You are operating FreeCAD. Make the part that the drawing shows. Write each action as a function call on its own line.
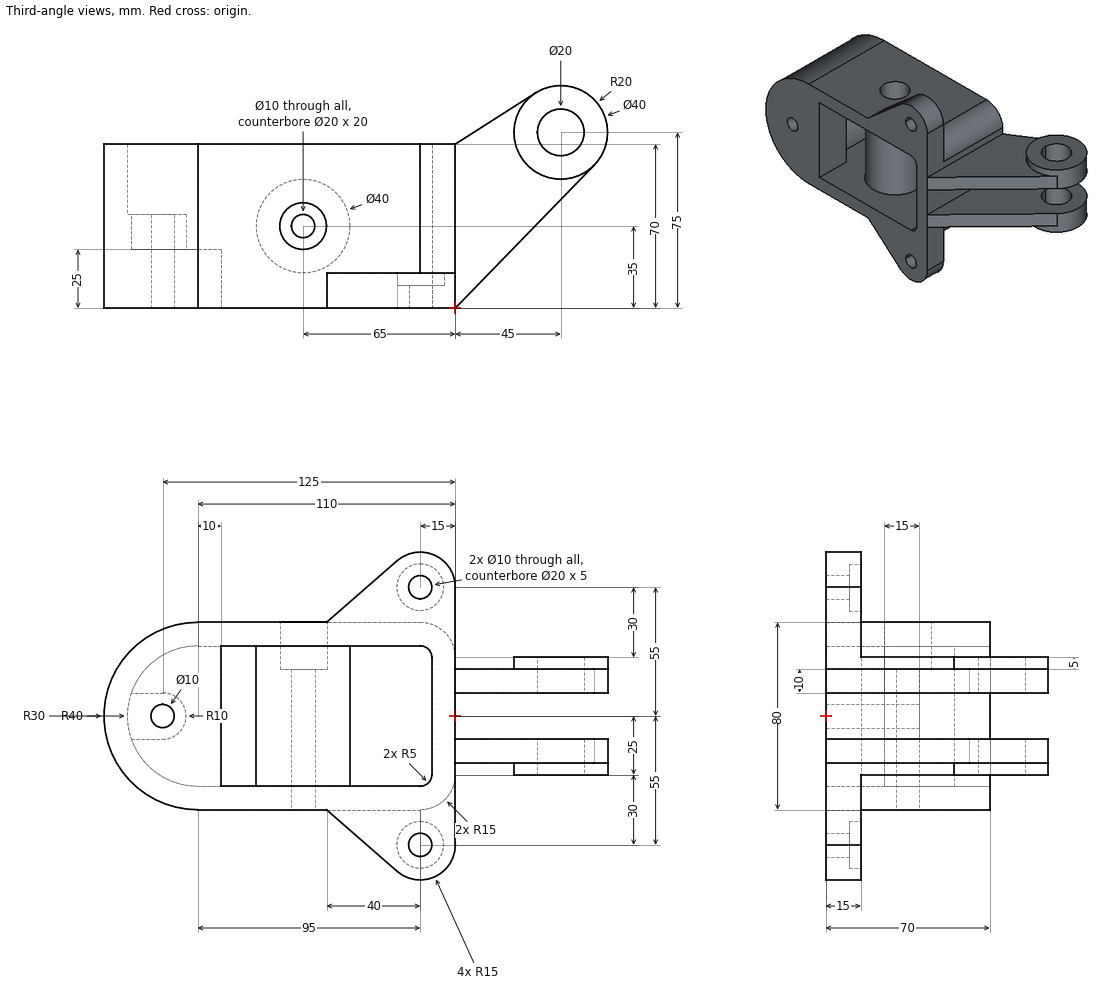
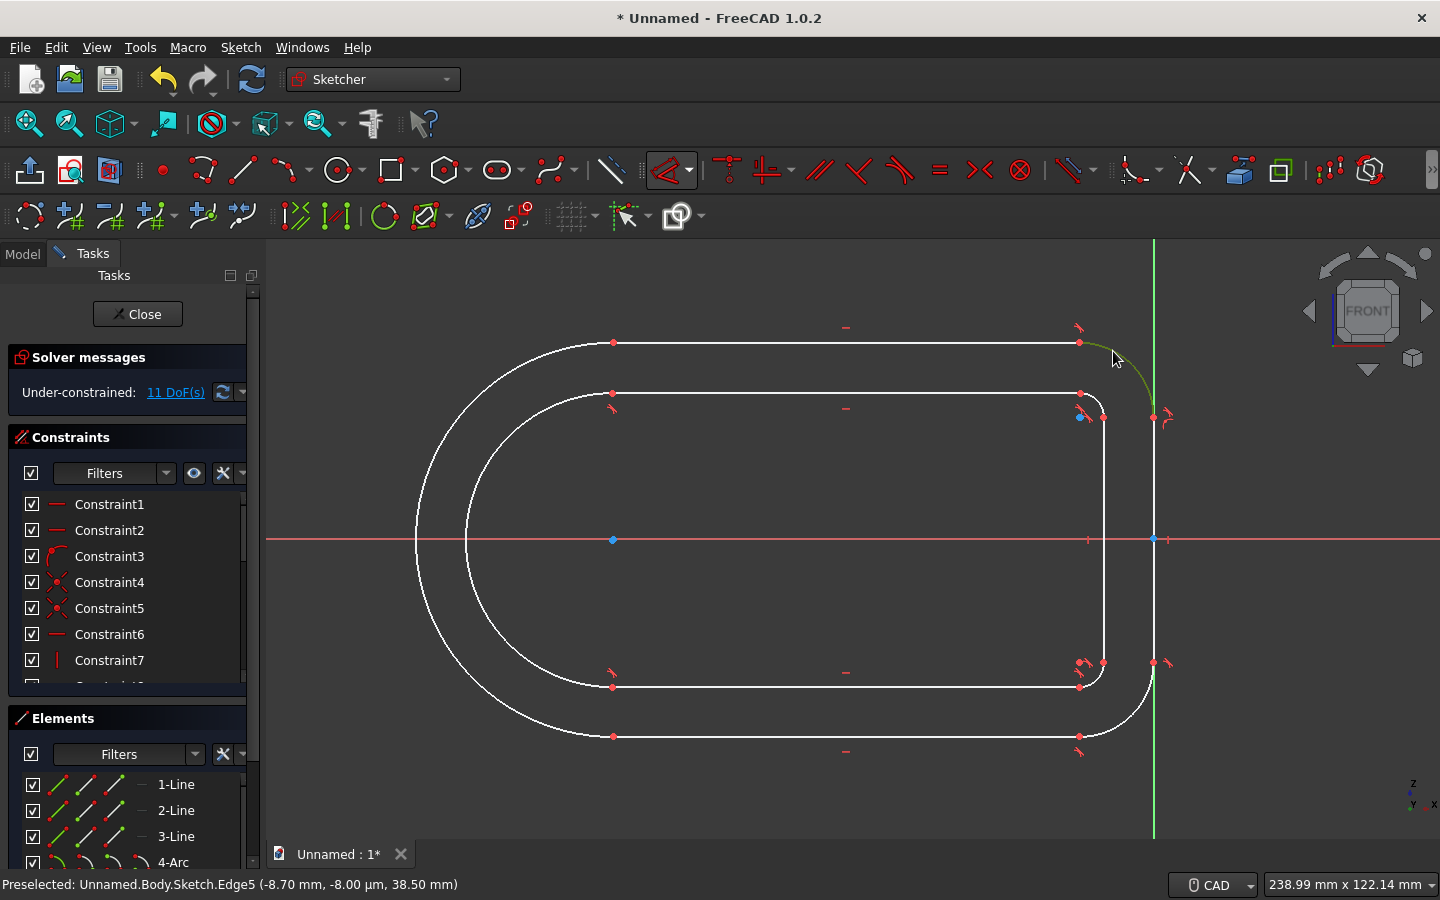
scroll(1101, 406, up, 2)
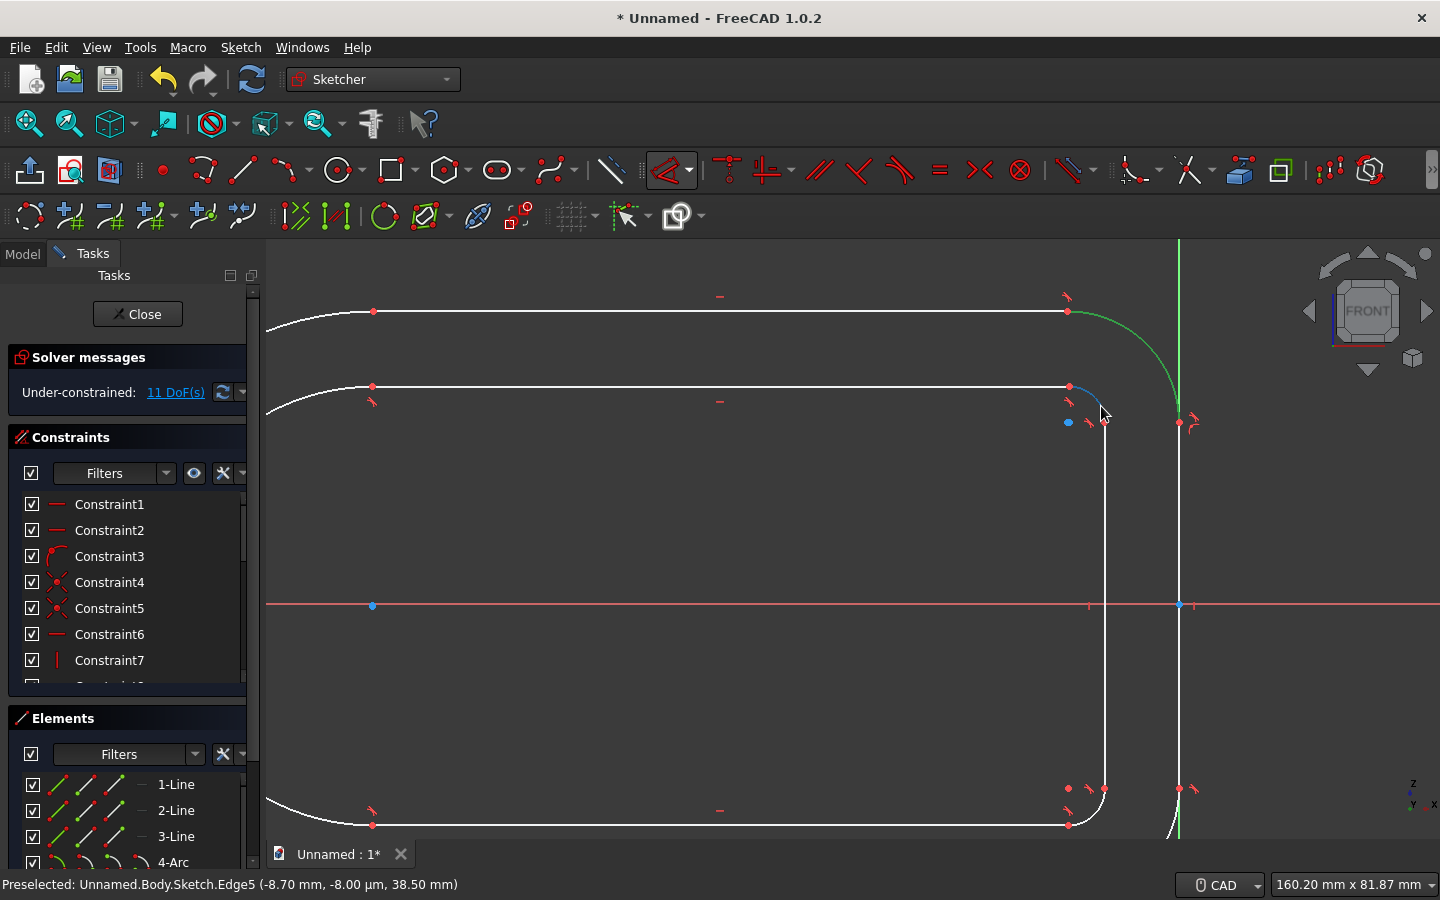
click(1101, 406)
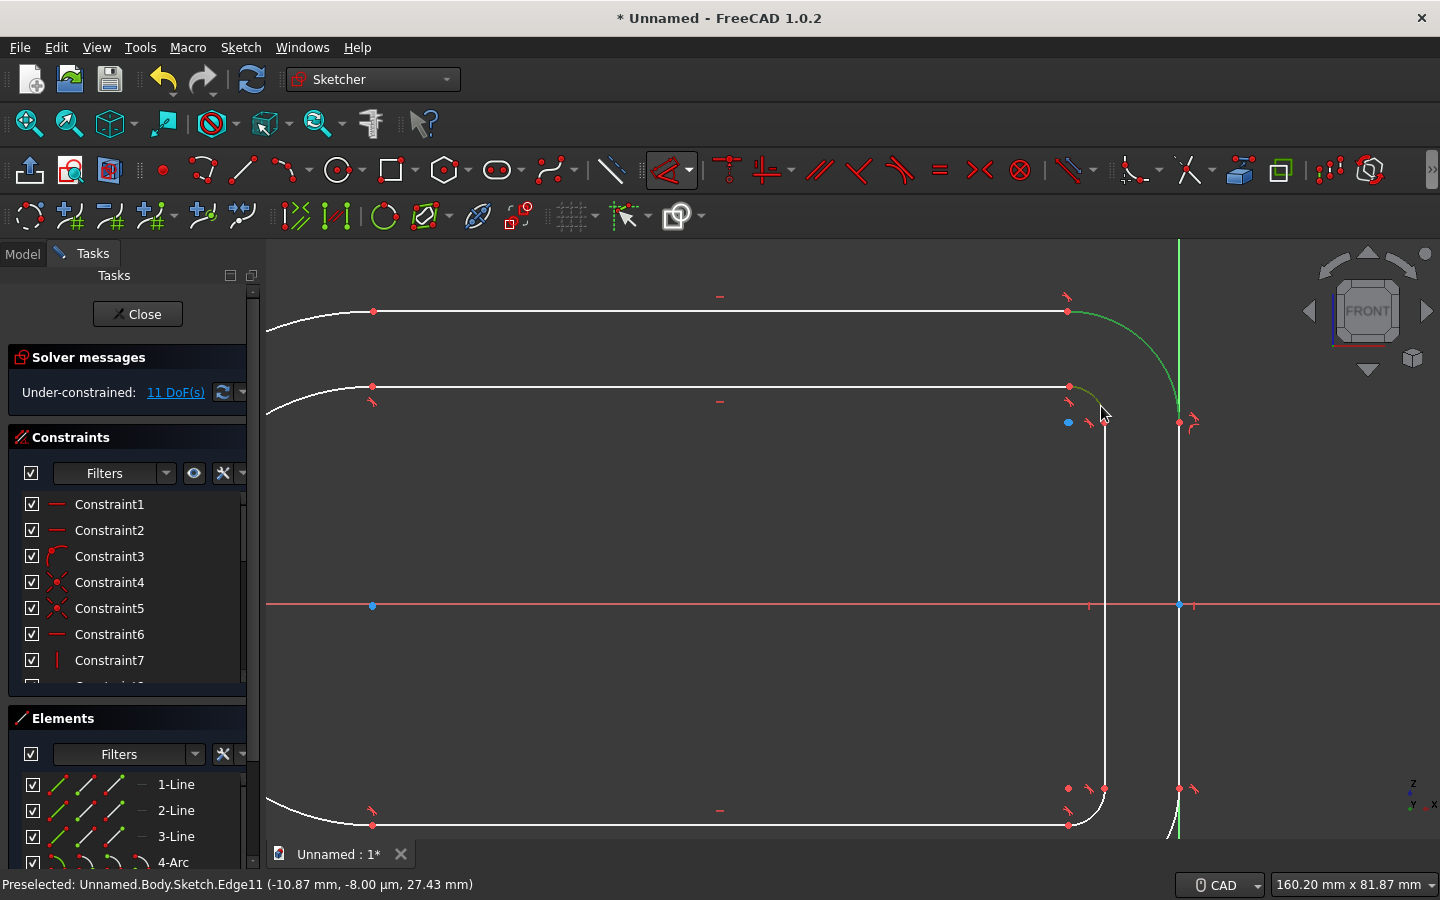
key(c)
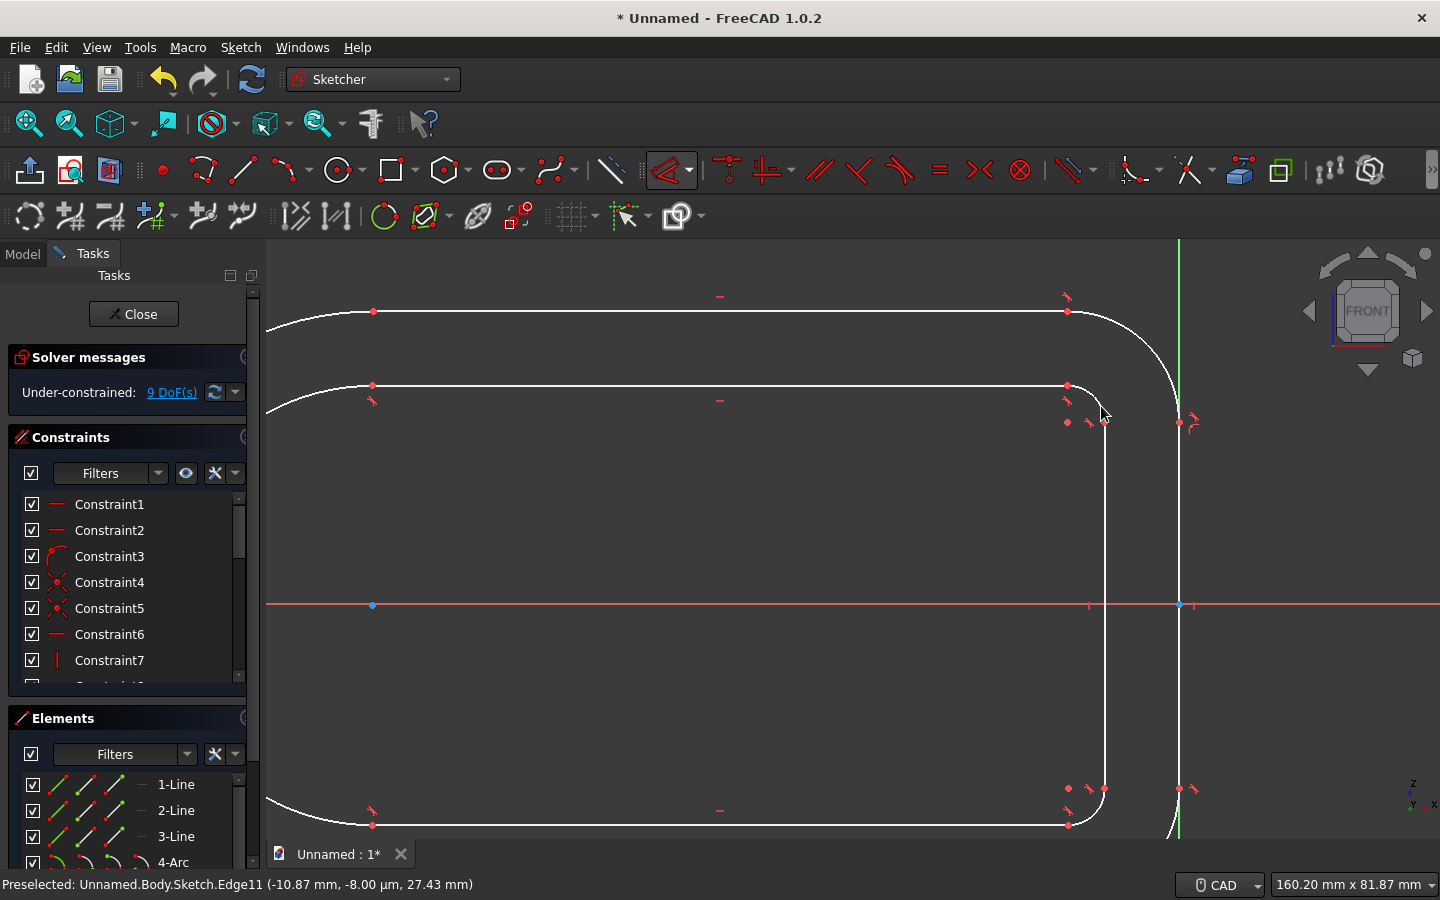
click(1167, 372)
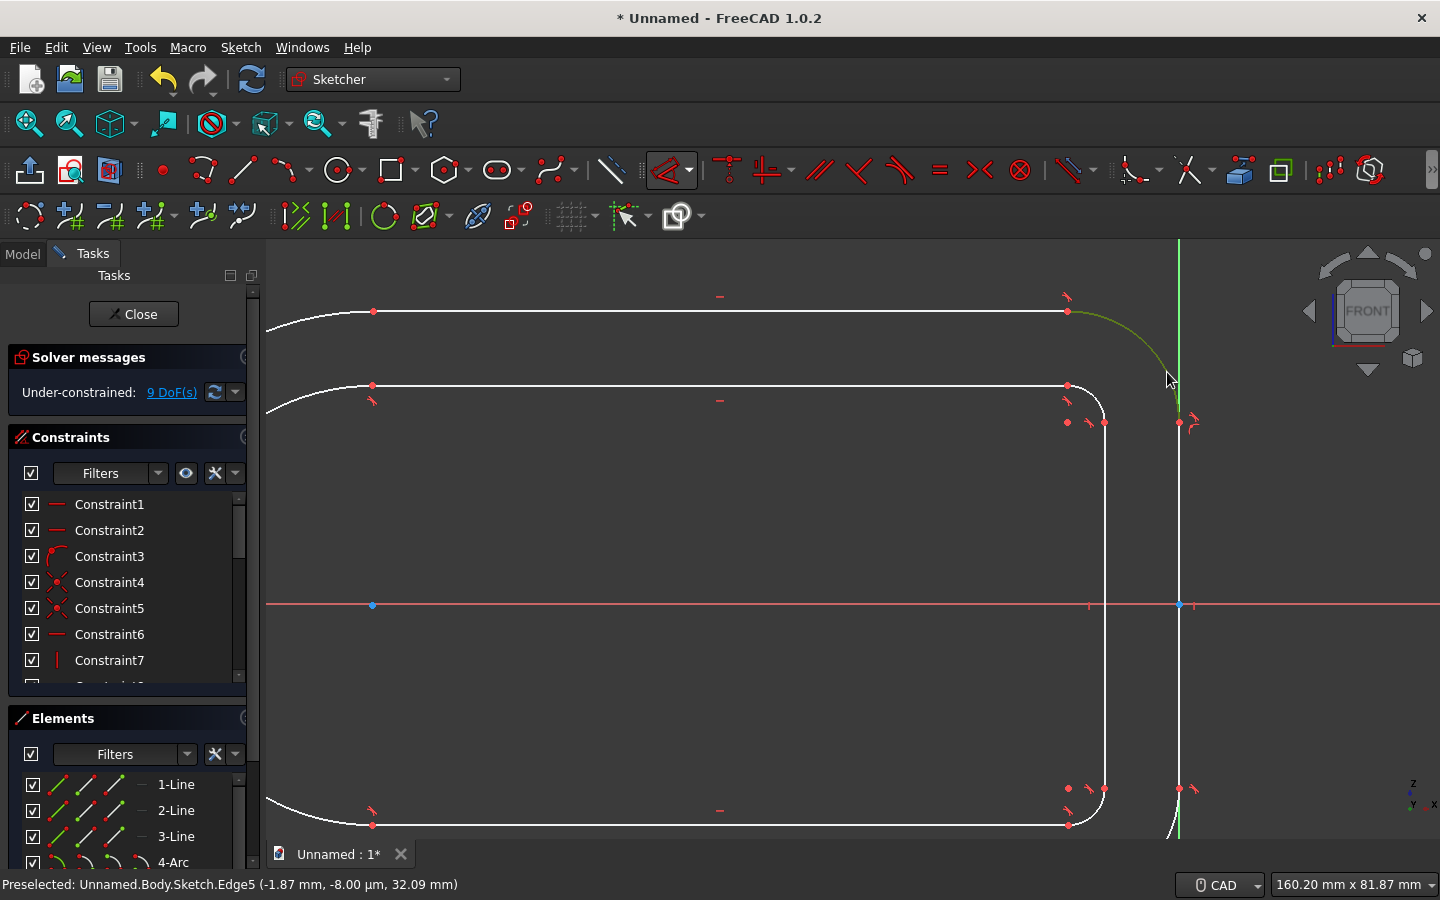
scroll(1100, 406, down, 2)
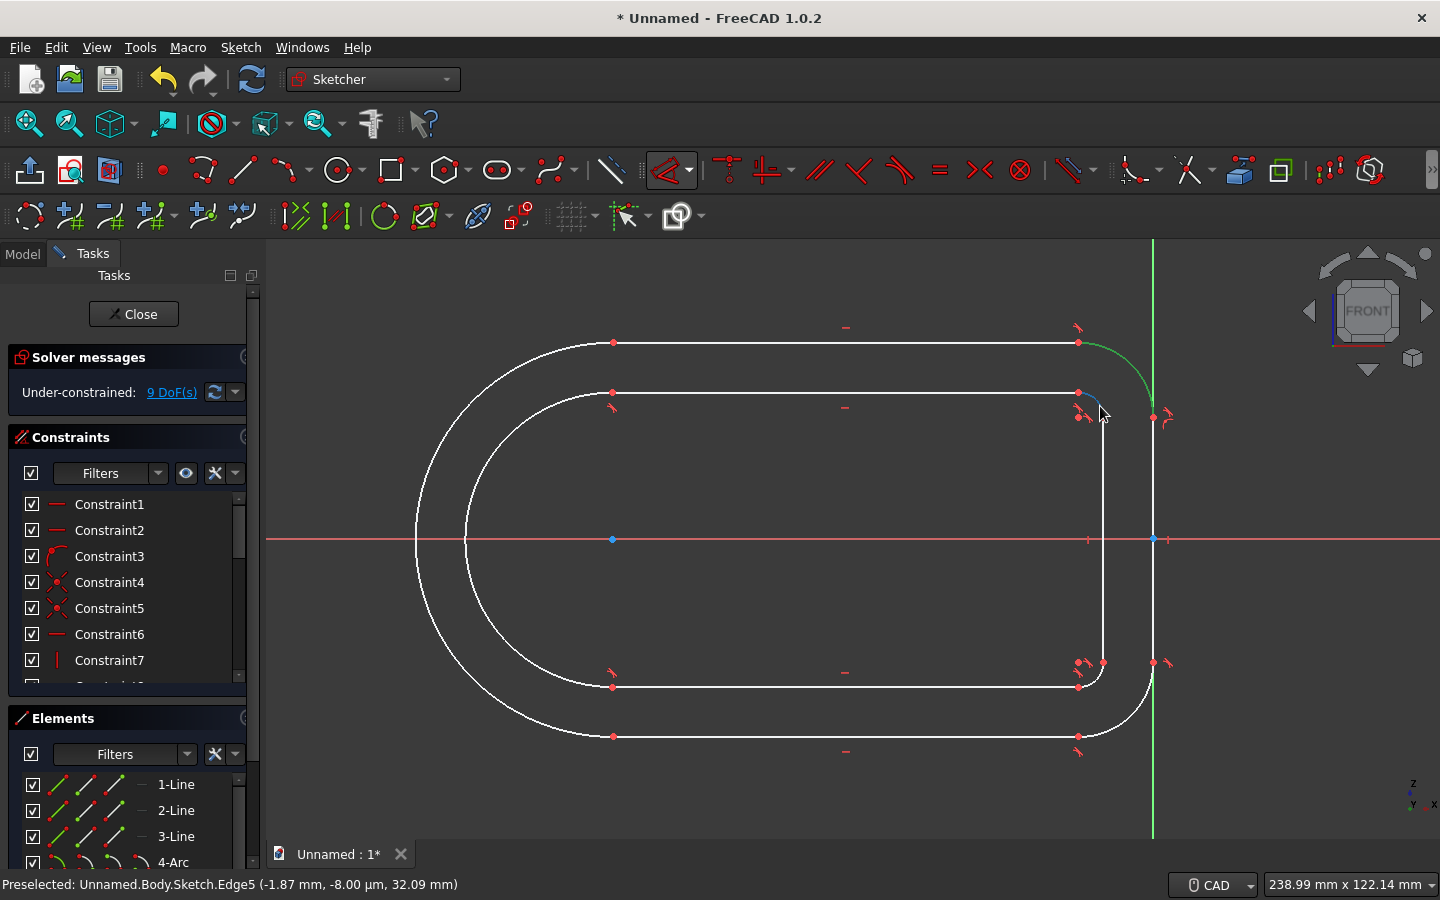
click(1113, 729)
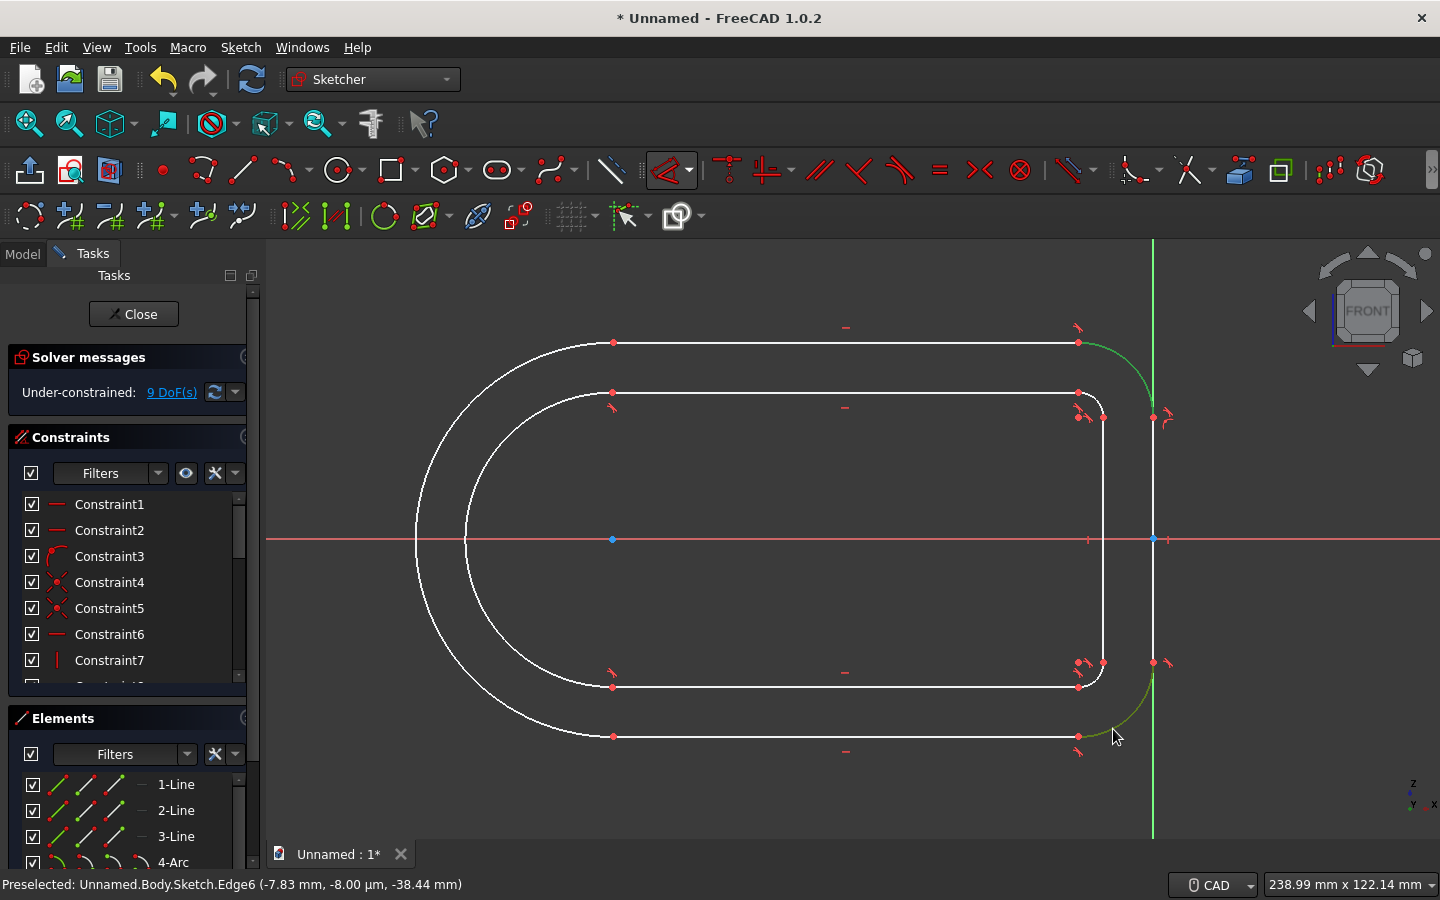
key(e)